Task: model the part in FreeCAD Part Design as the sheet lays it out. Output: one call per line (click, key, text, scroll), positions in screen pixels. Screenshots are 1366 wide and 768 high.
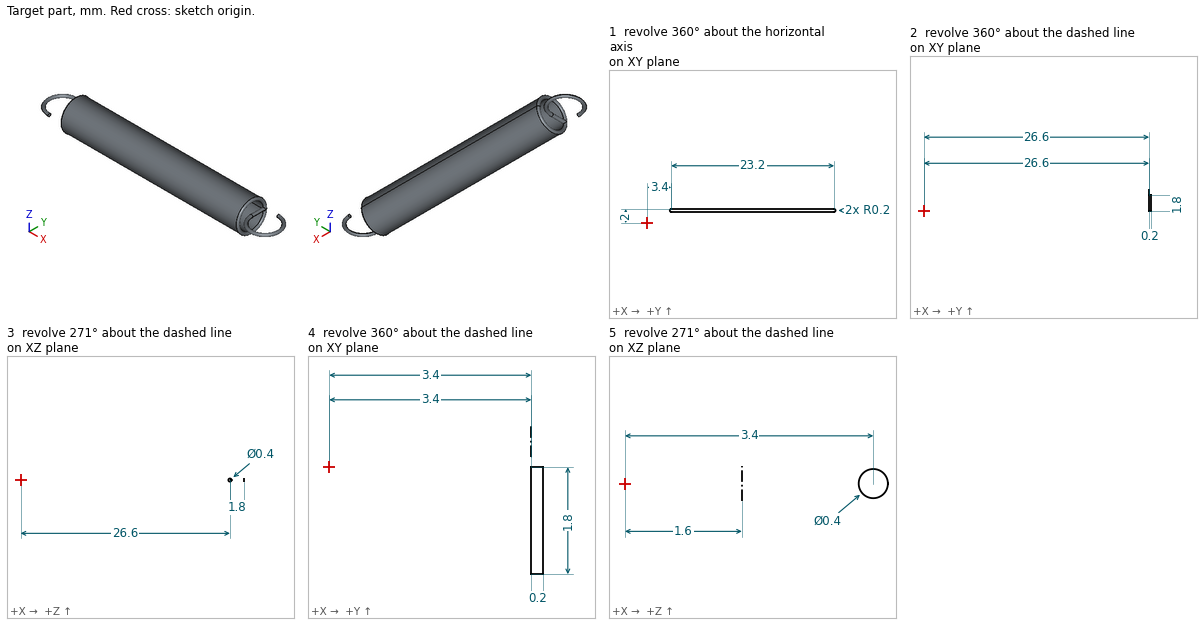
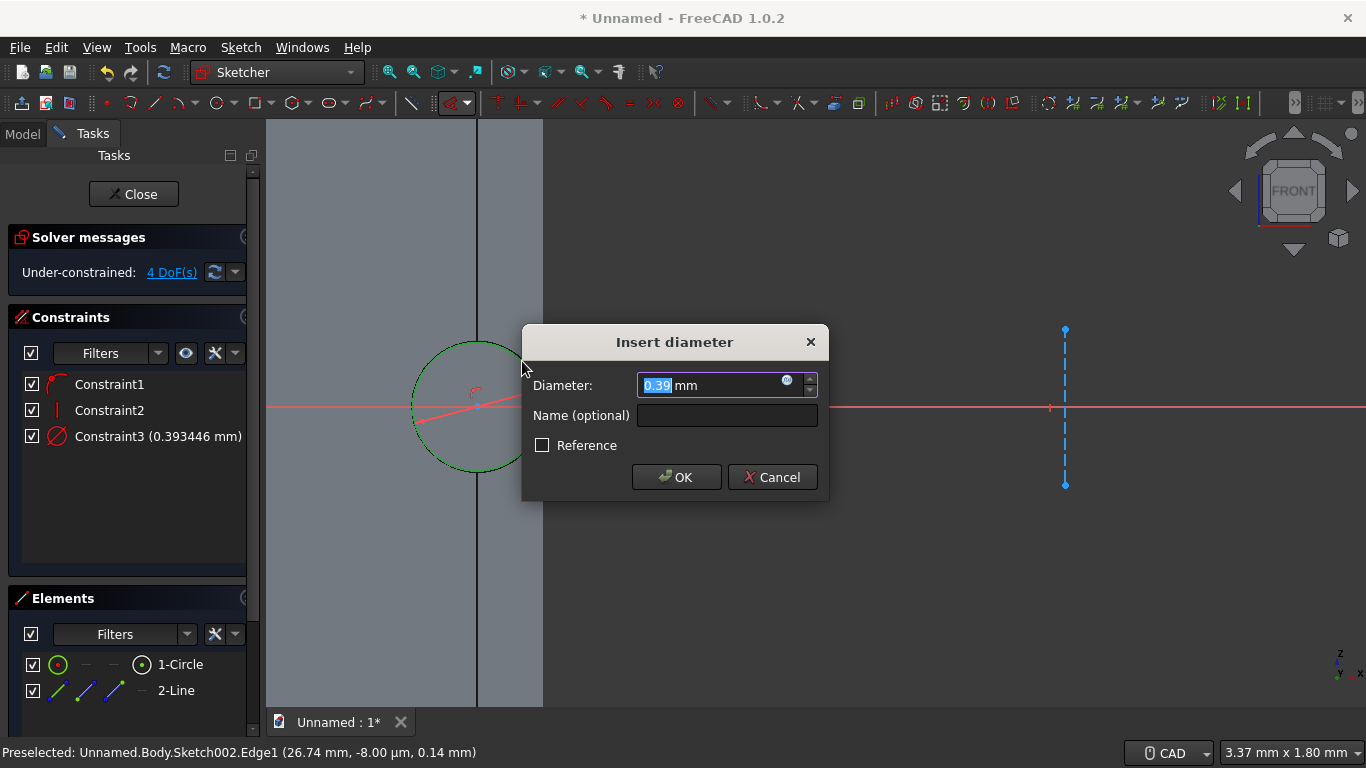
text(0.4)
key(Return)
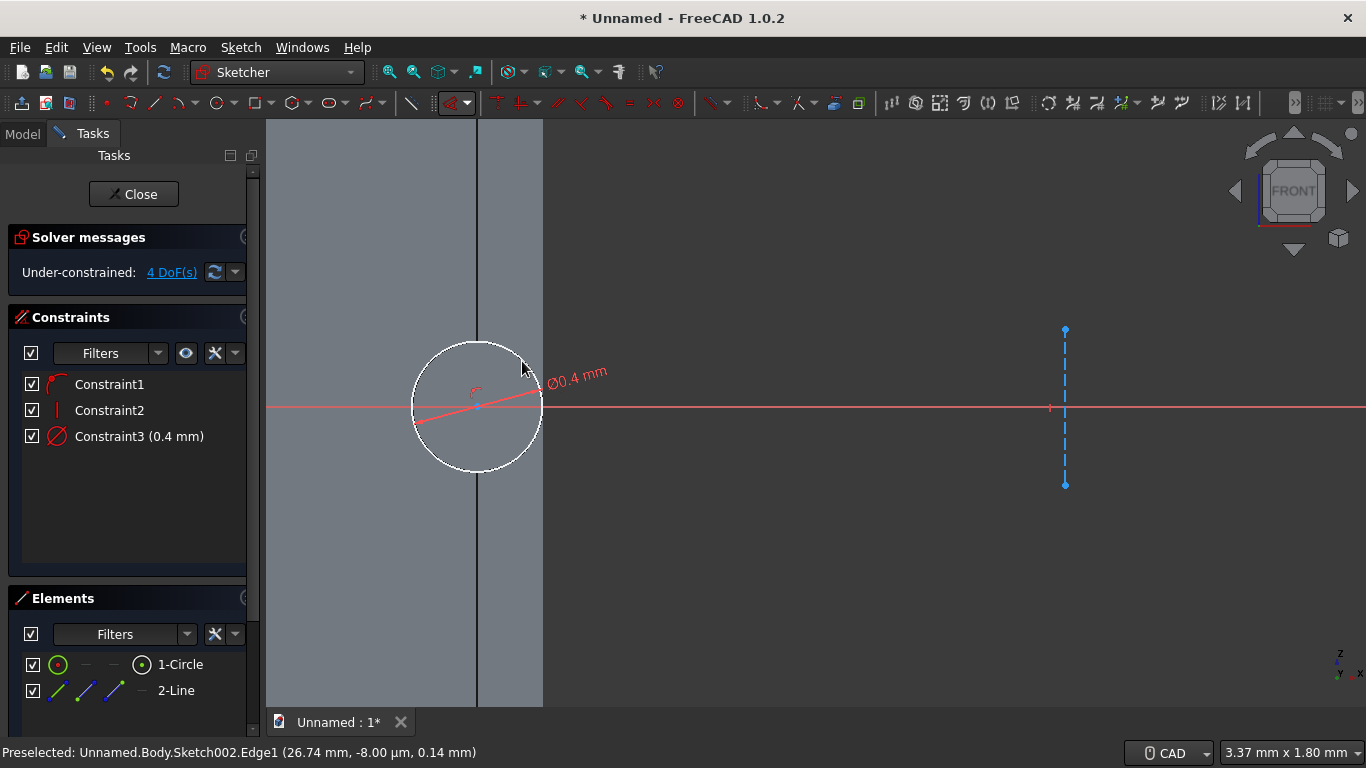
click(477, 407)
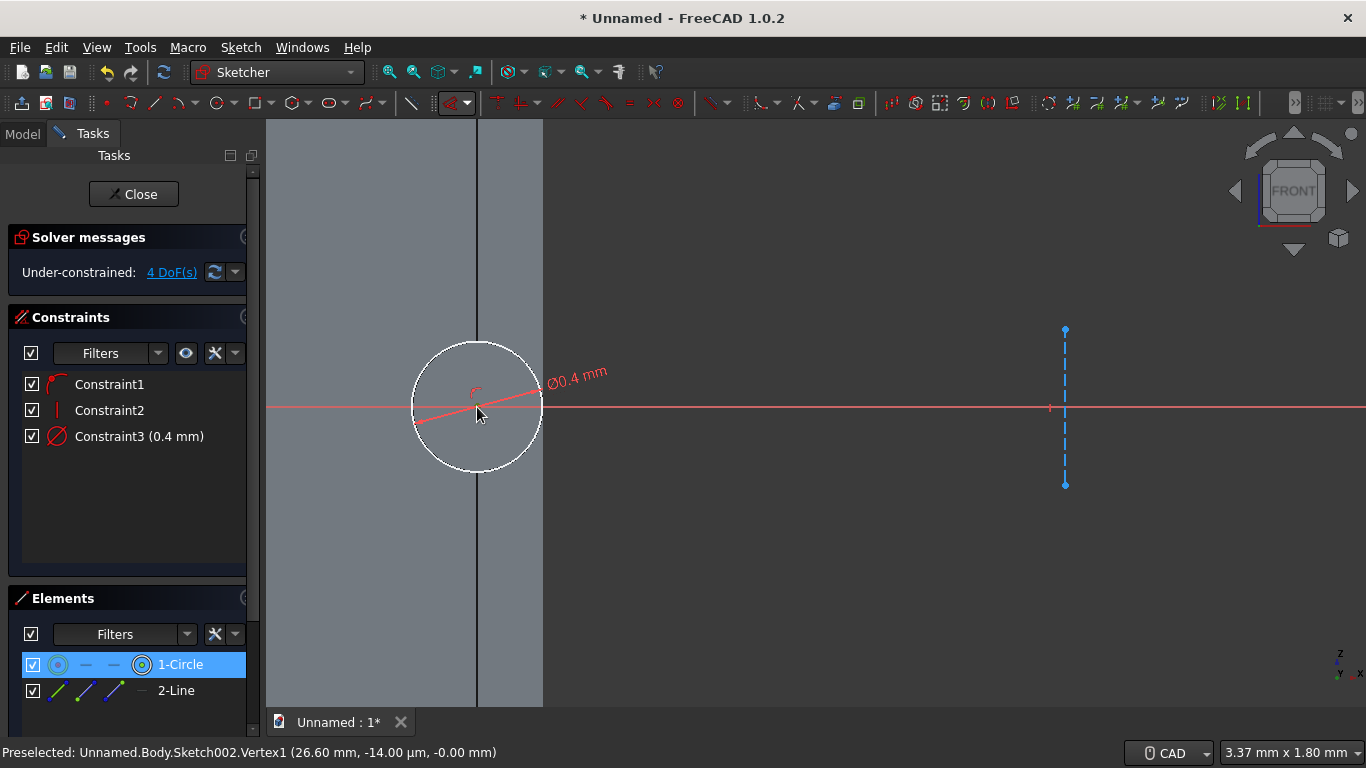
key(l)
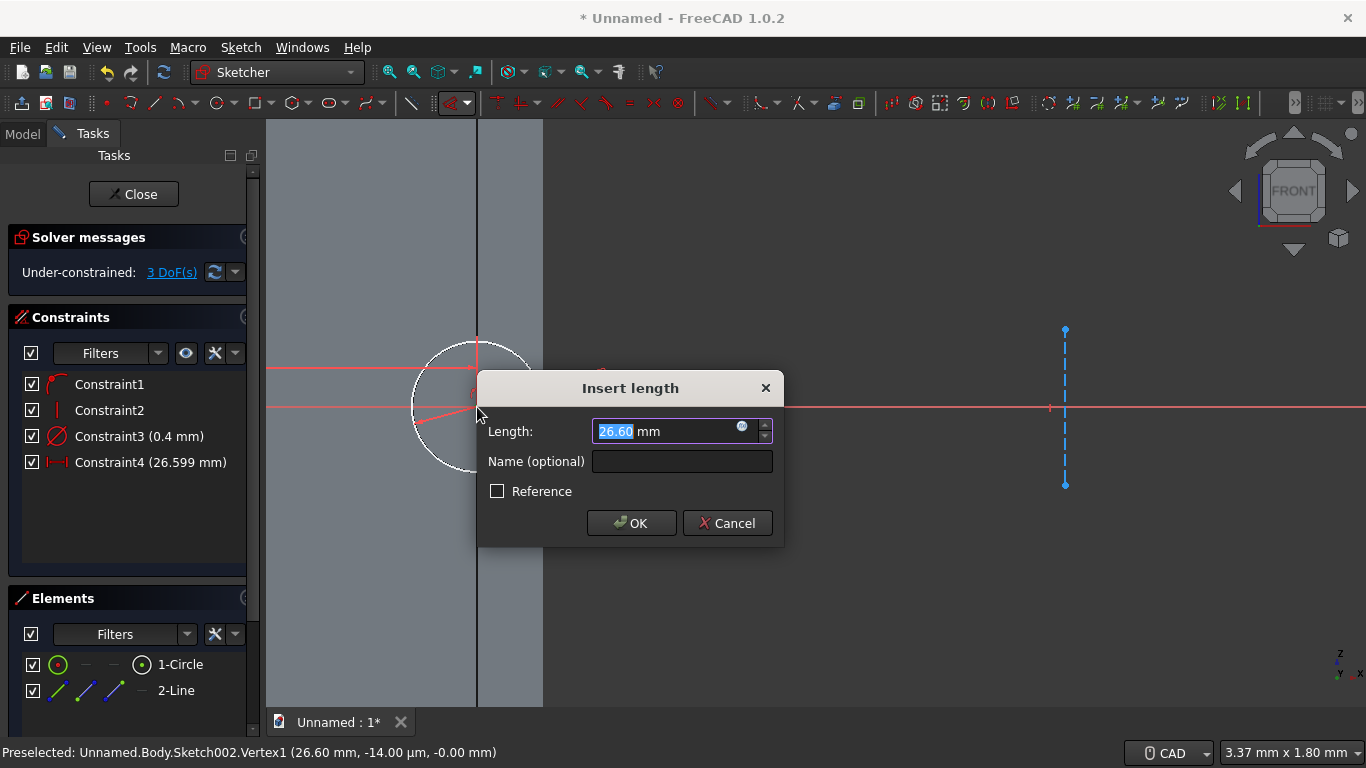
text(26.6)
key(Return)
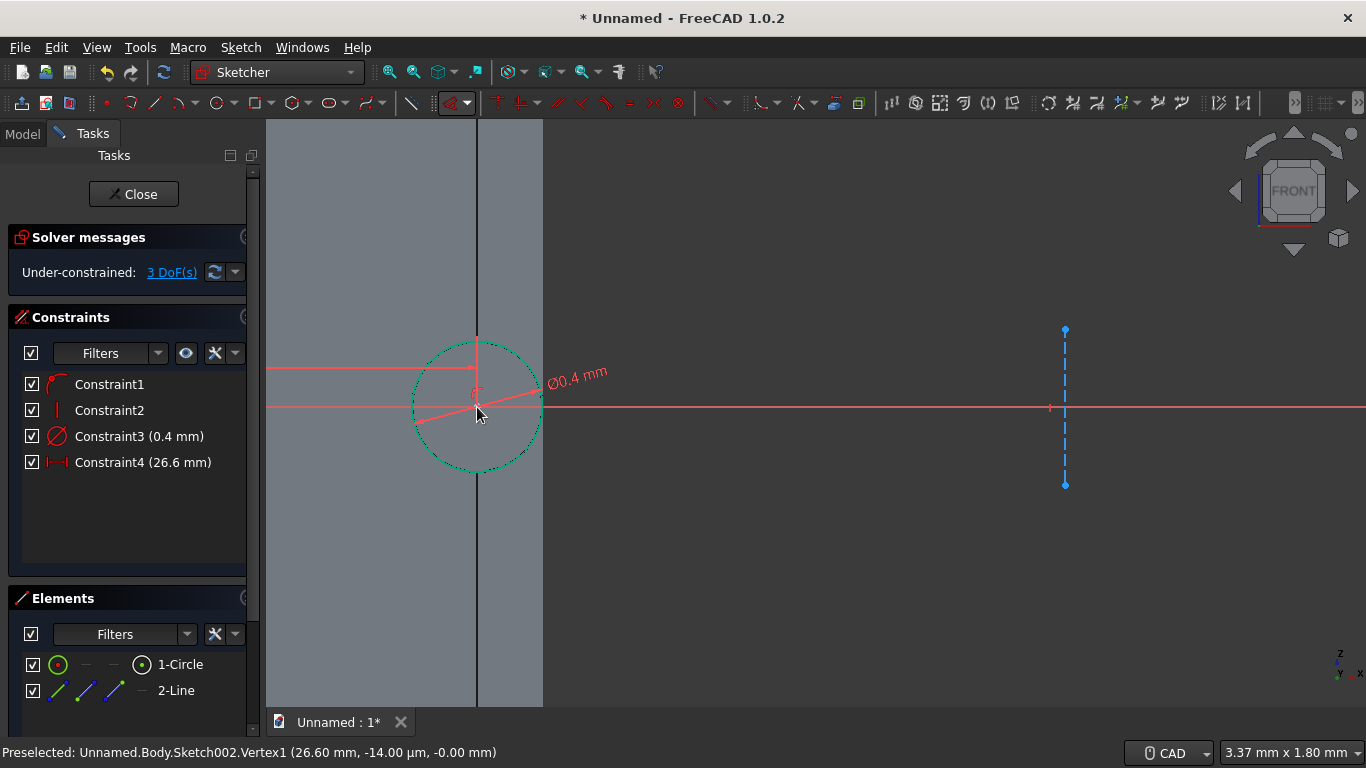
click(1065, 486)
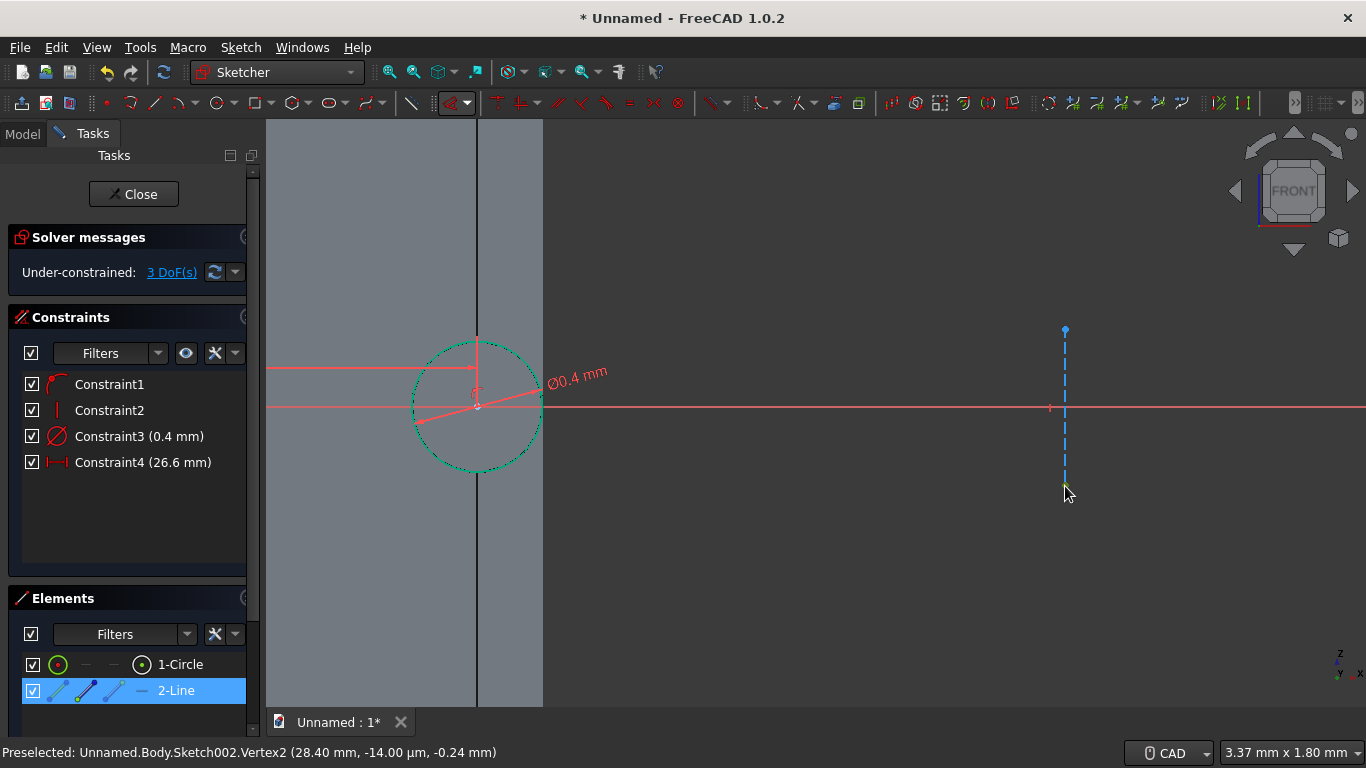
click(477, 407)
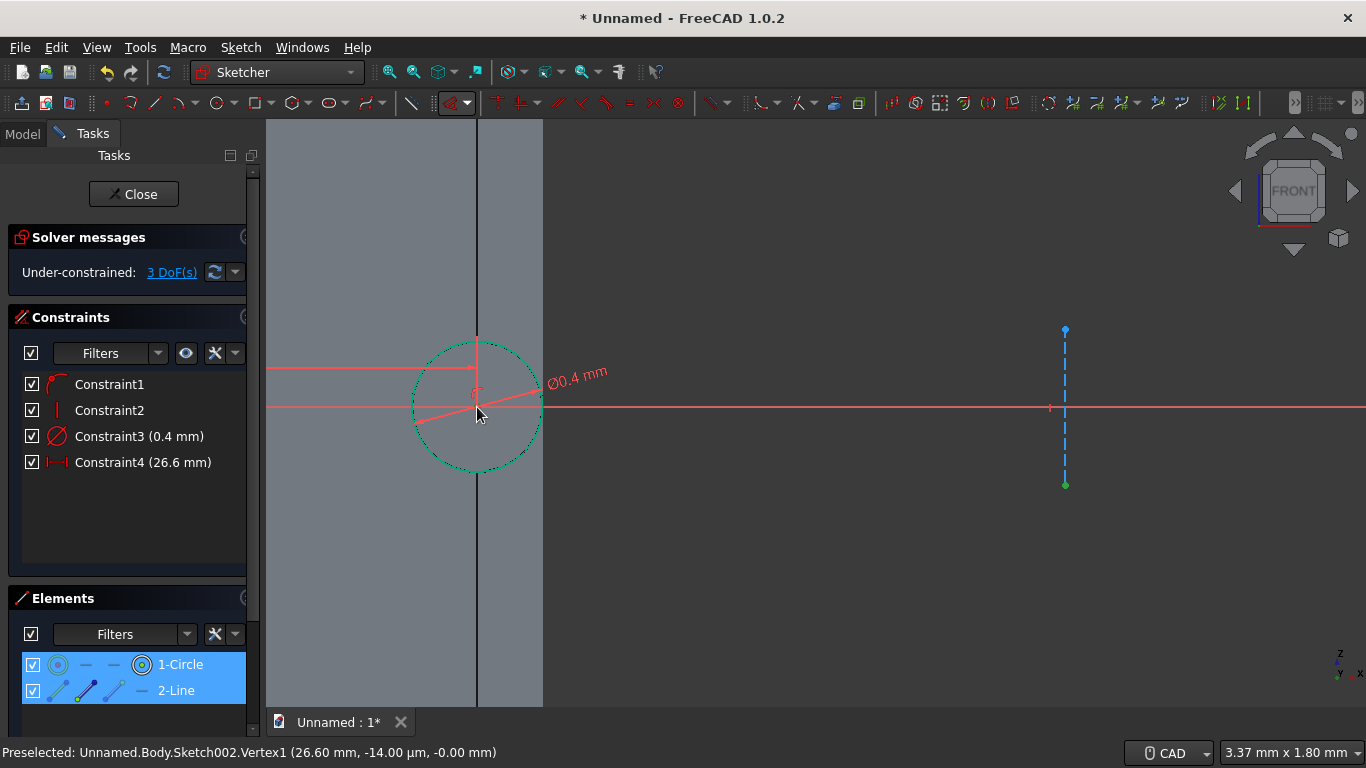
key(l)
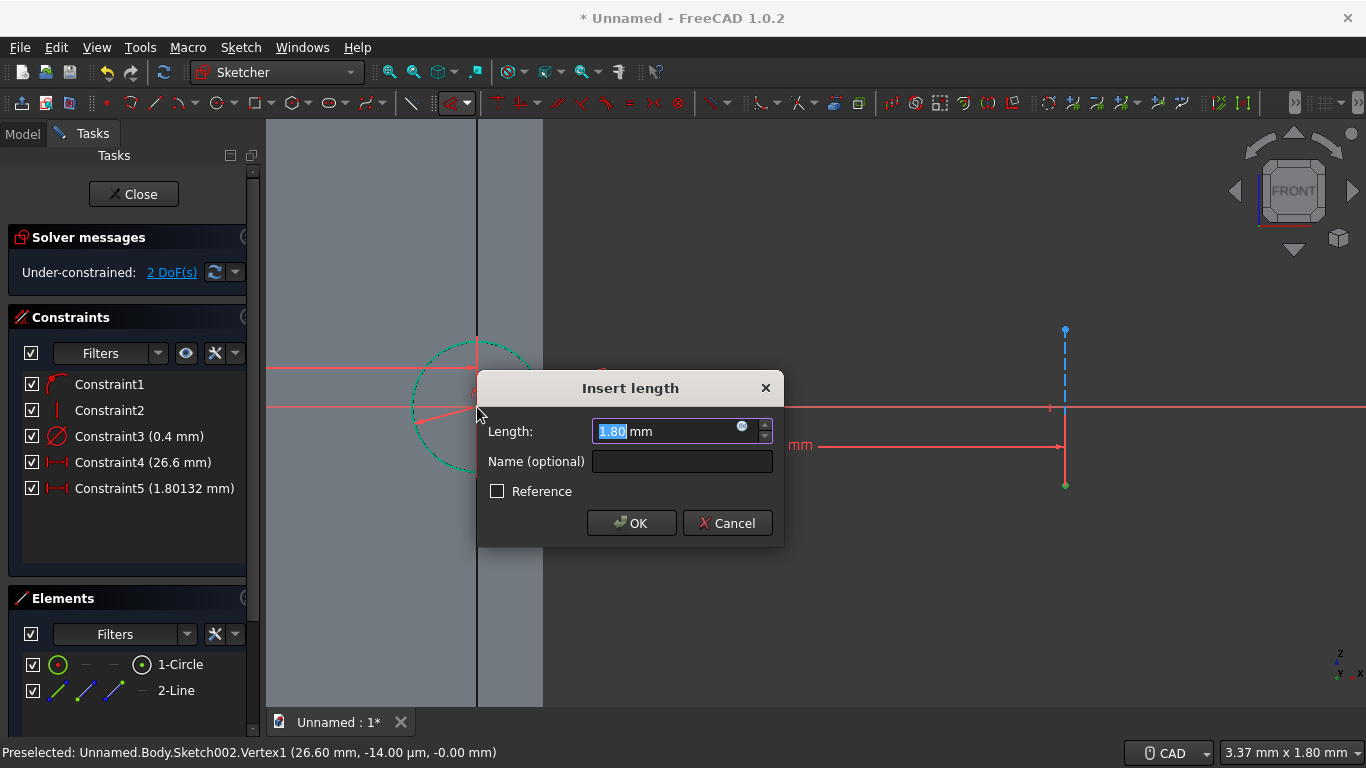
text(1.8)
key(Return)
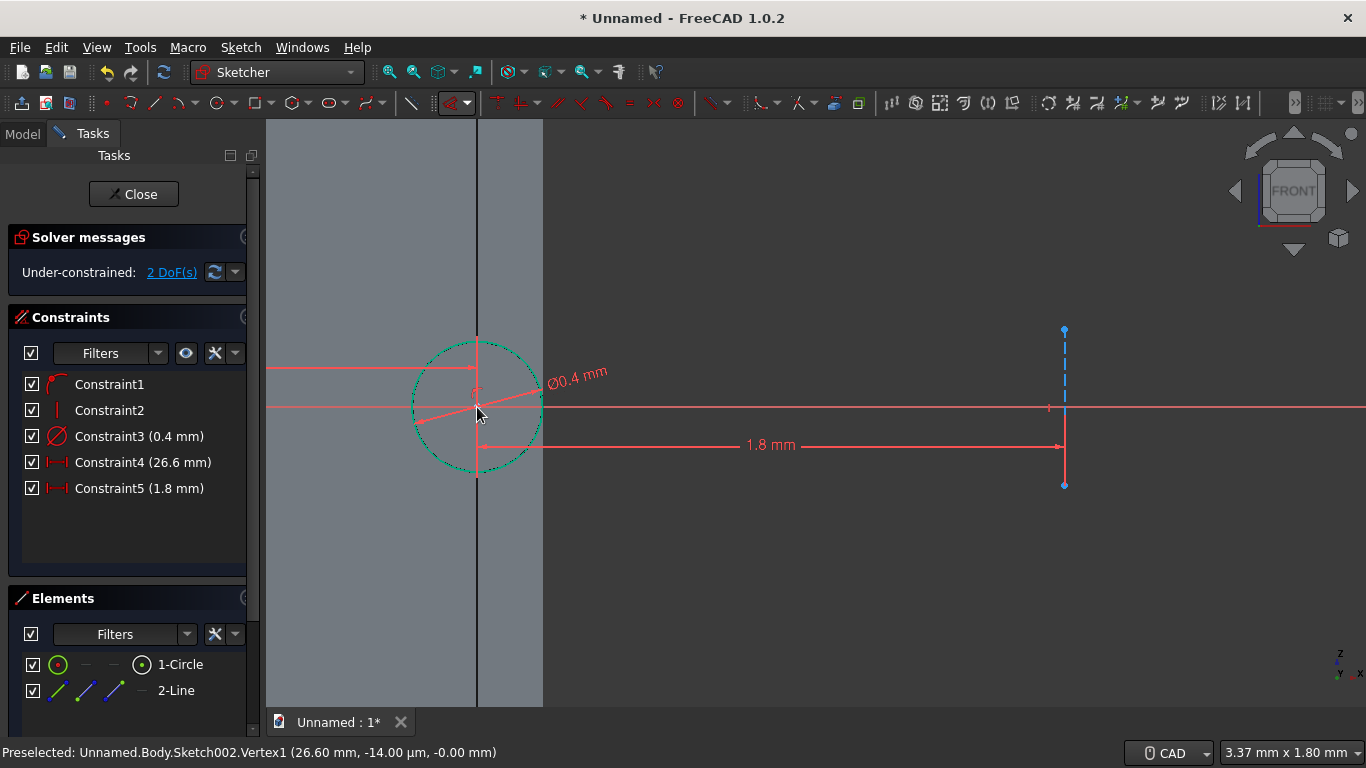
click(134, 194)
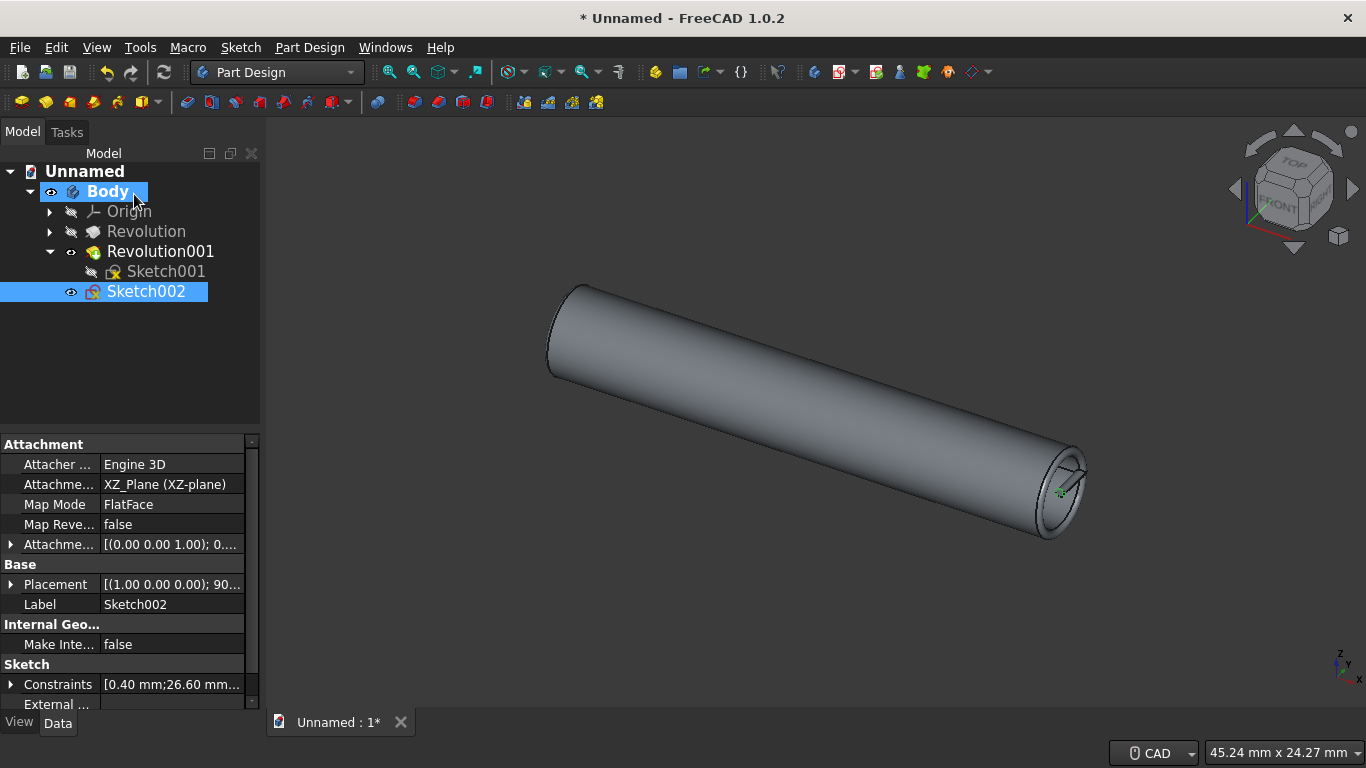
click(46, 102)